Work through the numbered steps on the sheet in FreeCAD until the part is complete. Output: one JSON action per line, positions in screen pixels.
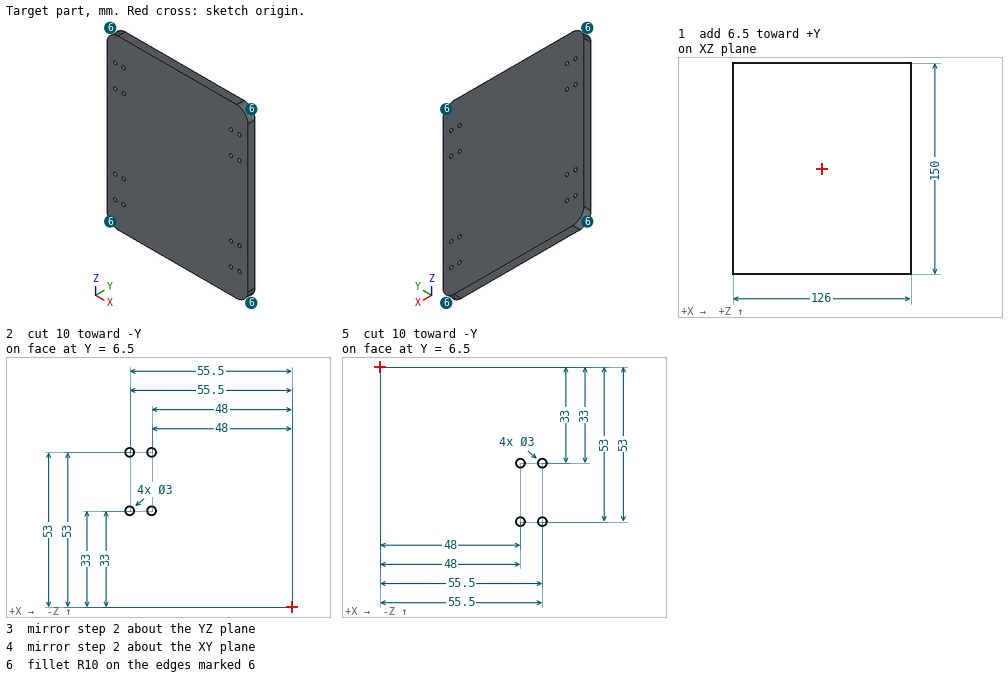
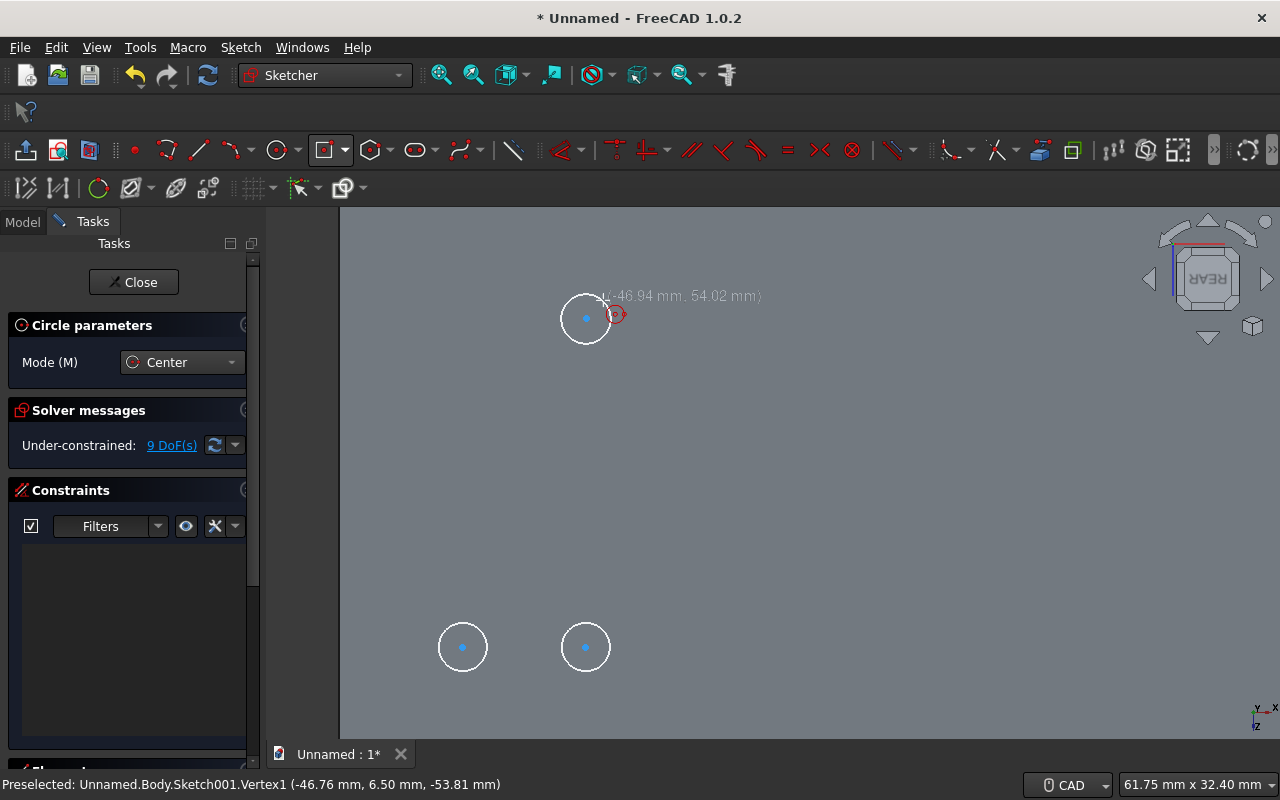
{"action": "left_click", "coordinate": [463, 318]}
{"action": "left_click", "coordinate": [480, 300]}
{"action": "key", "text": "Escape"}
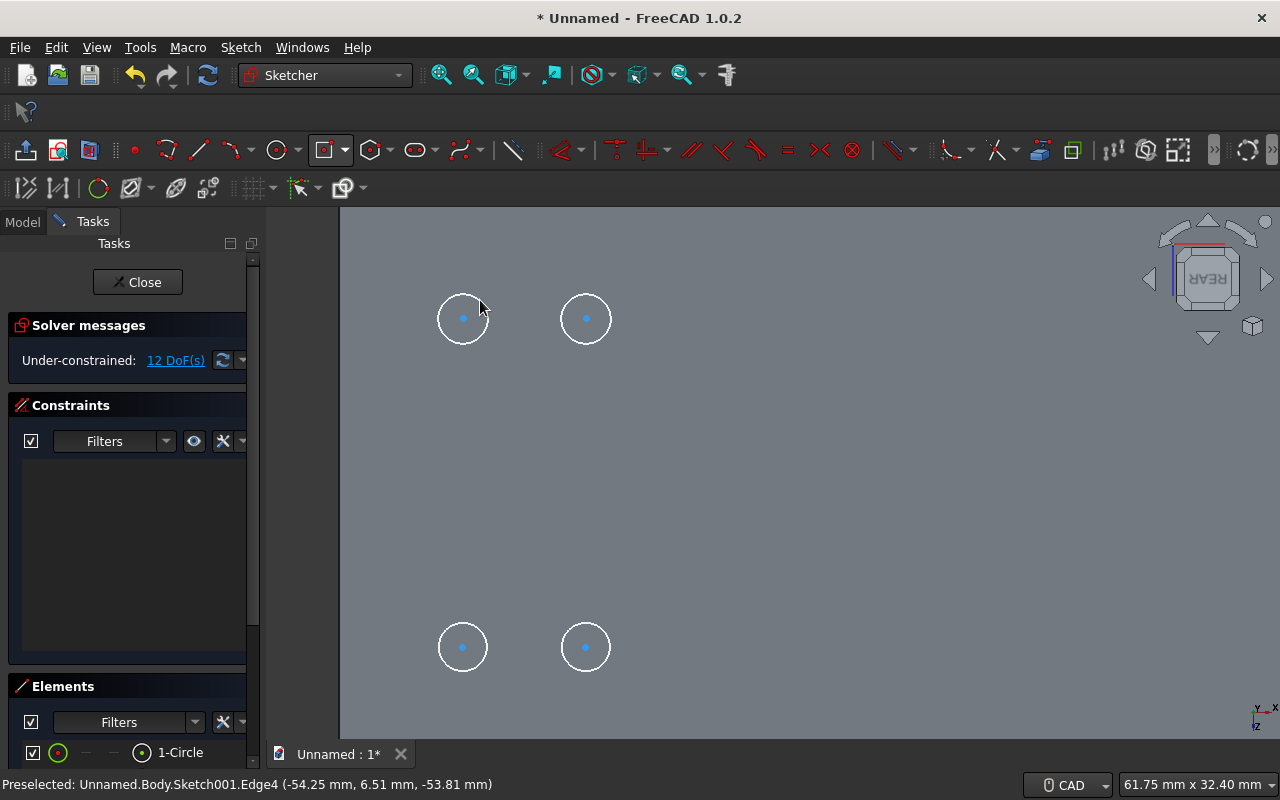
{"action": "left_click", "coordinate": [480, 630]}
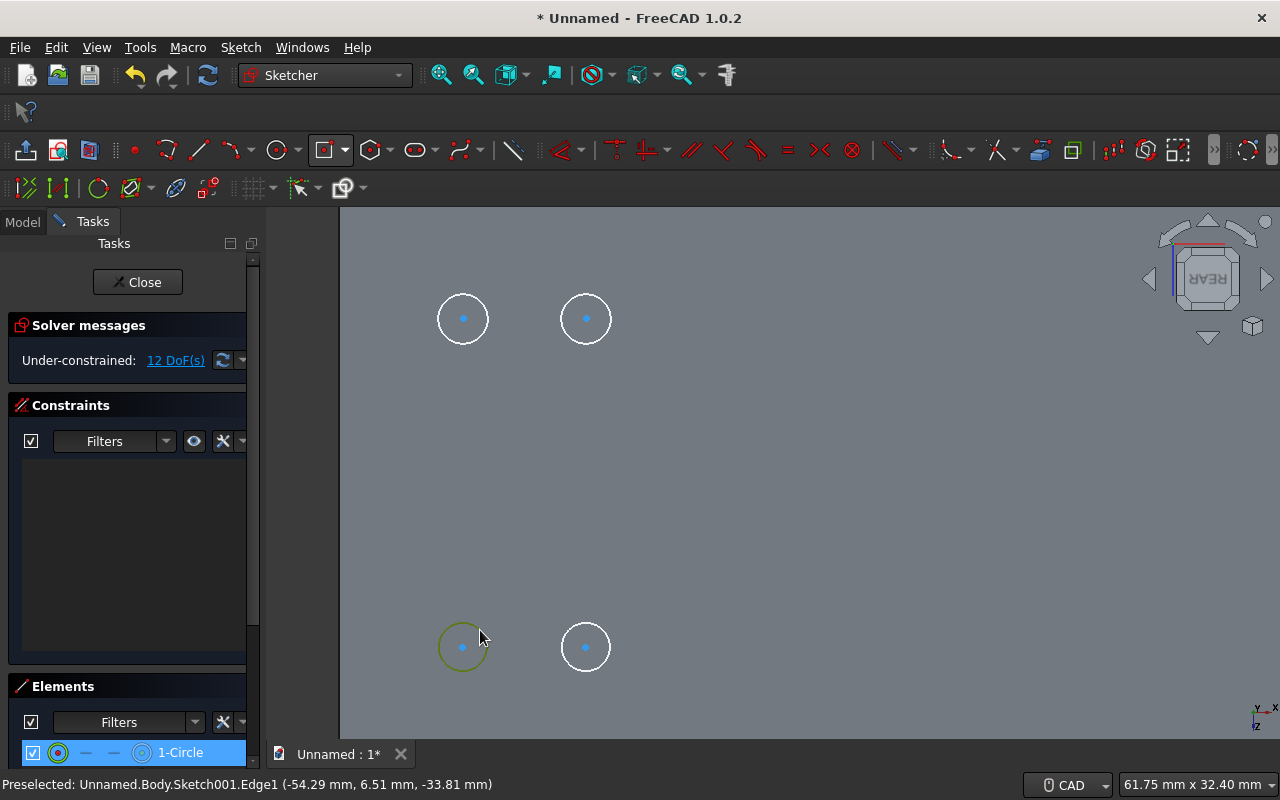
{"action": "left_click", "coordinate": [603, 630]}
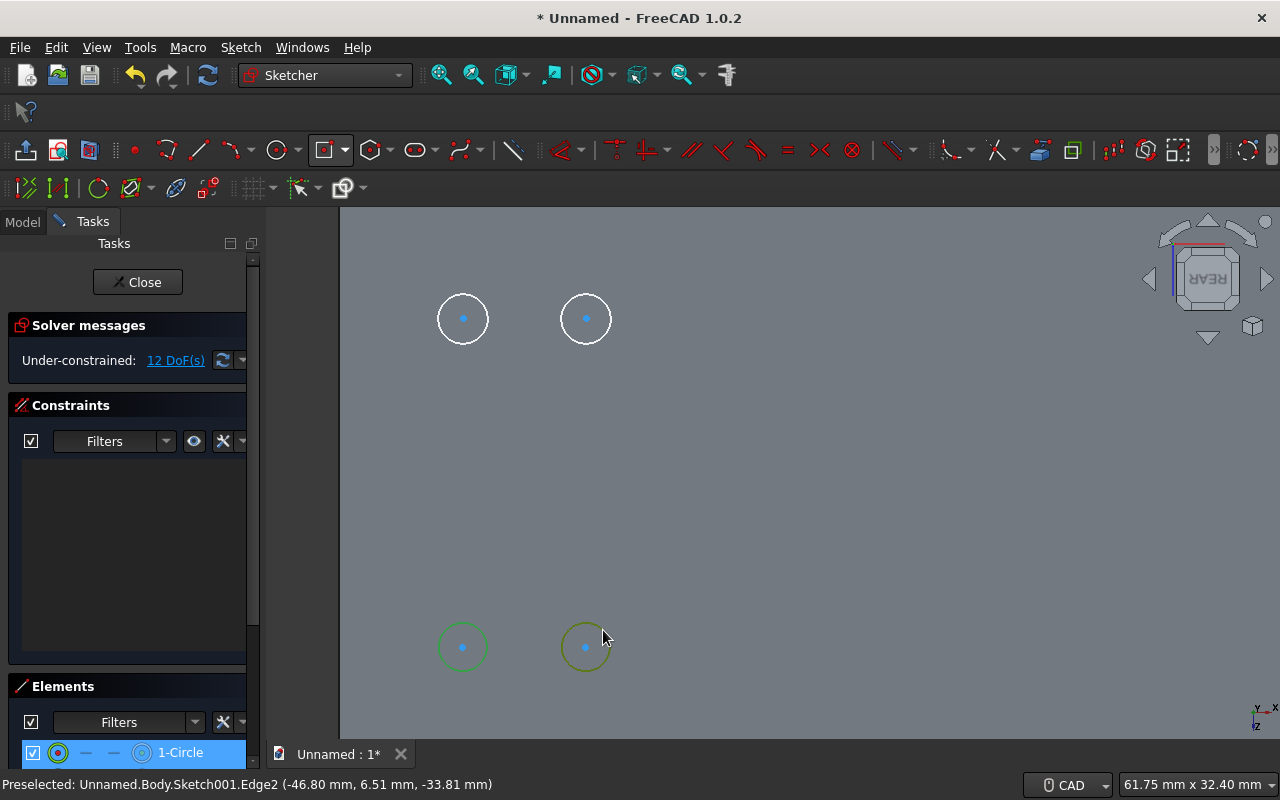
{"action": "left_click", "coordinate": [603, 301]}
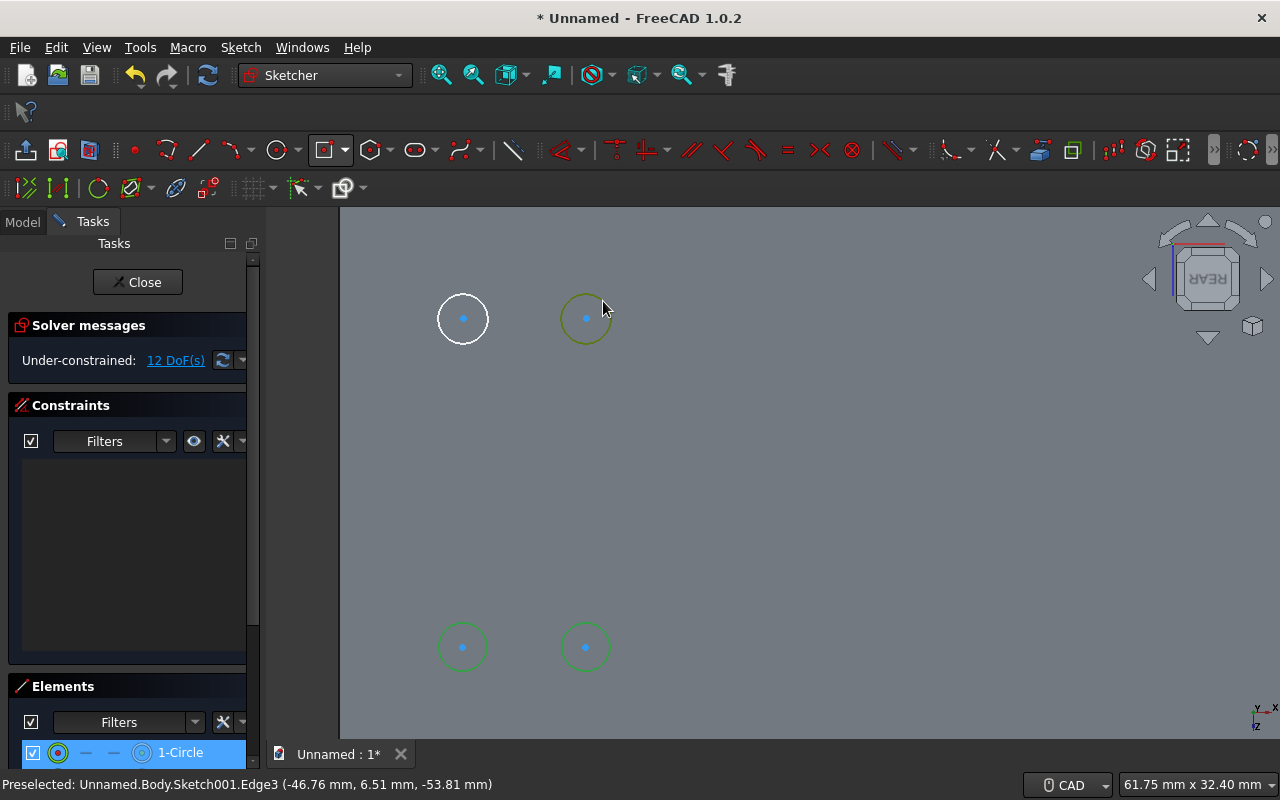
{"action": "left_click", "coordinate": [480, 301]}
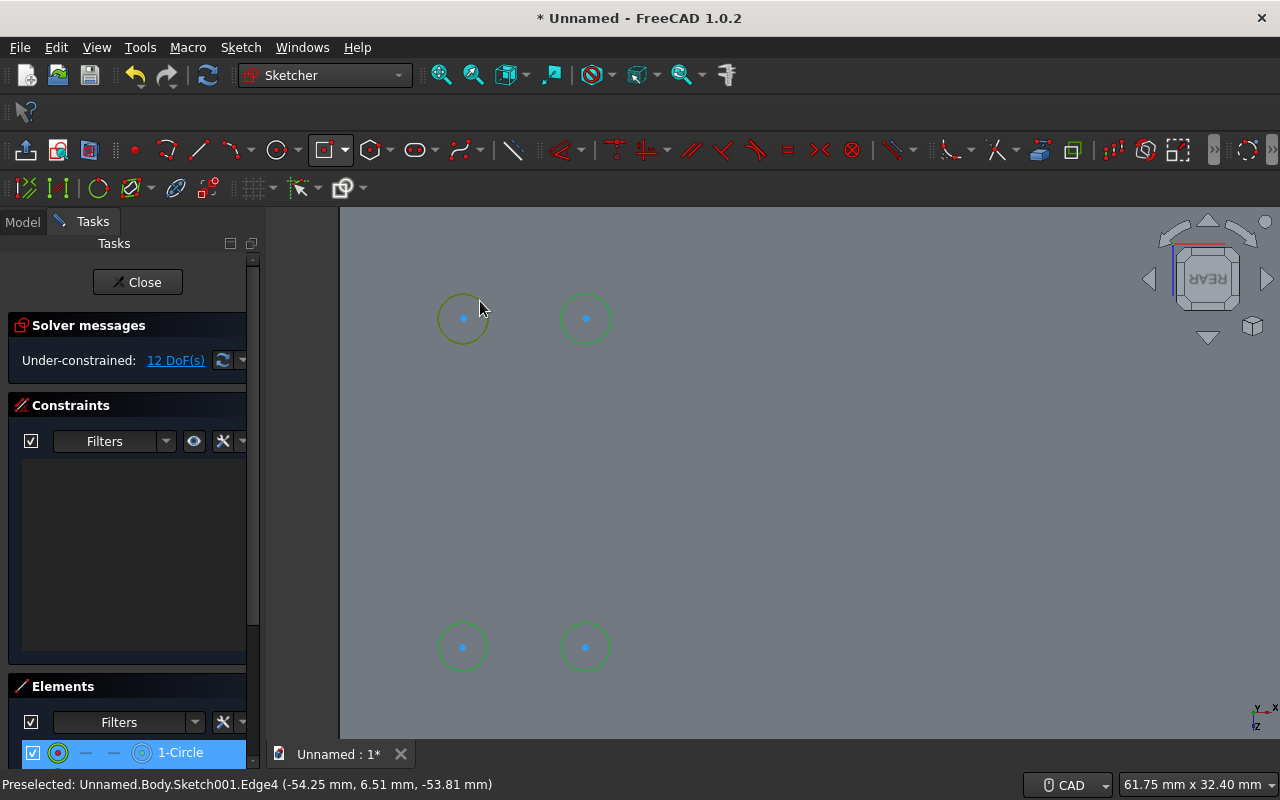
{"action": "key", "text": "e"}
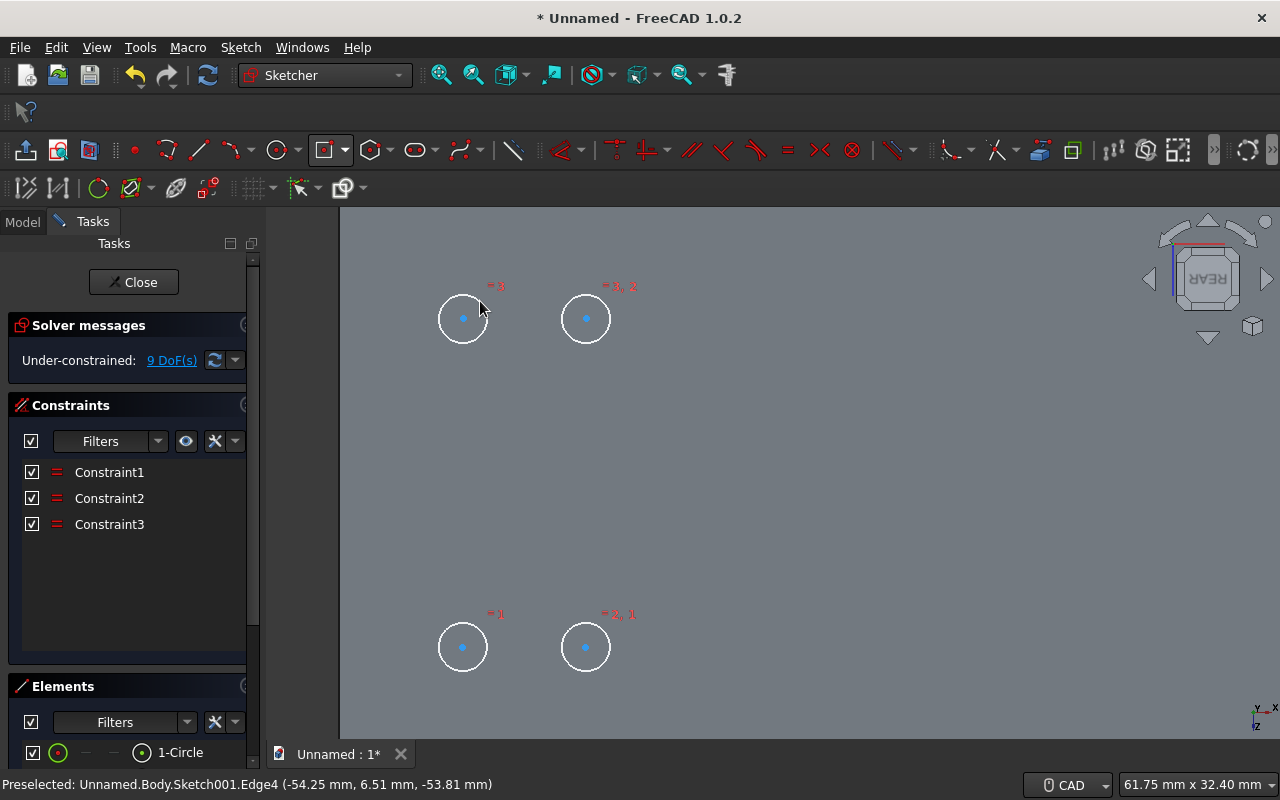
{"action": "left_click", "coordinate": [560, 150]}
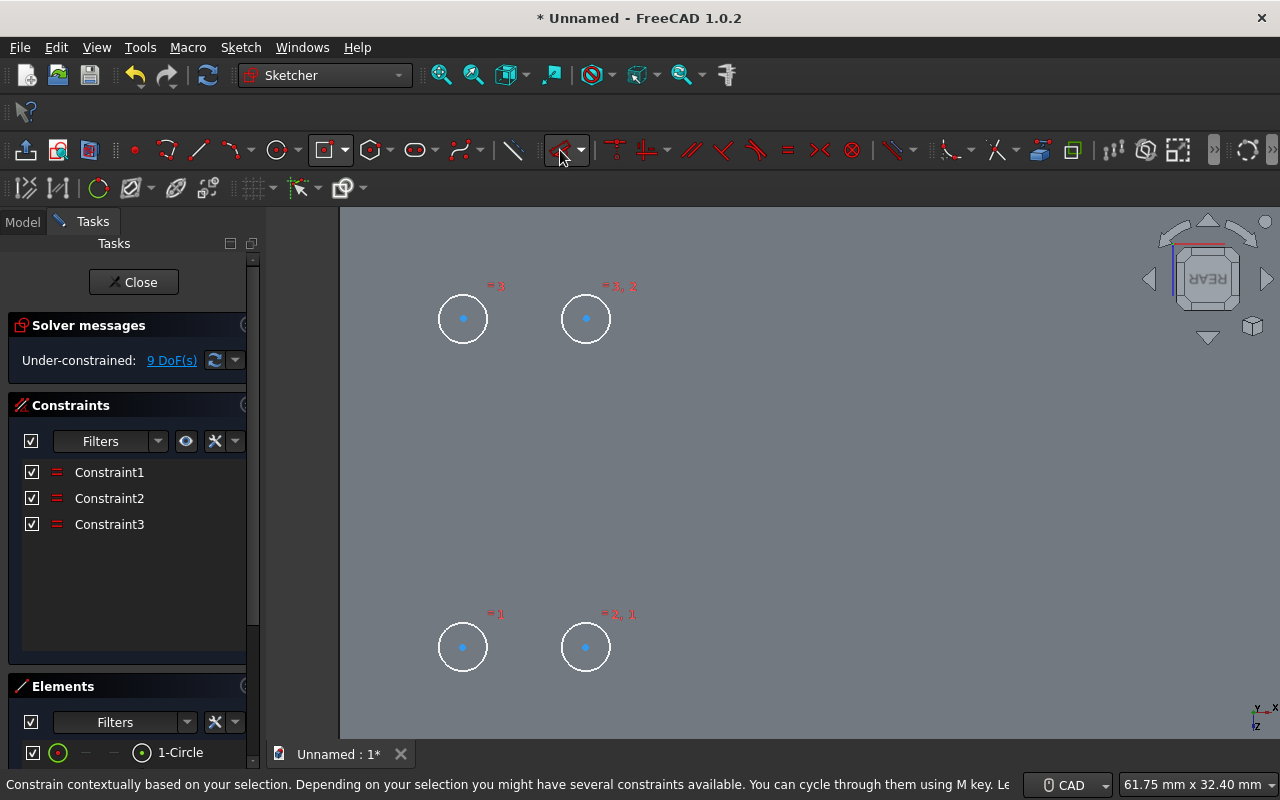
{"action": "left_click", "coordinate": [480, 630]}
{"action": "left_click", "coordinate": [503, 607]}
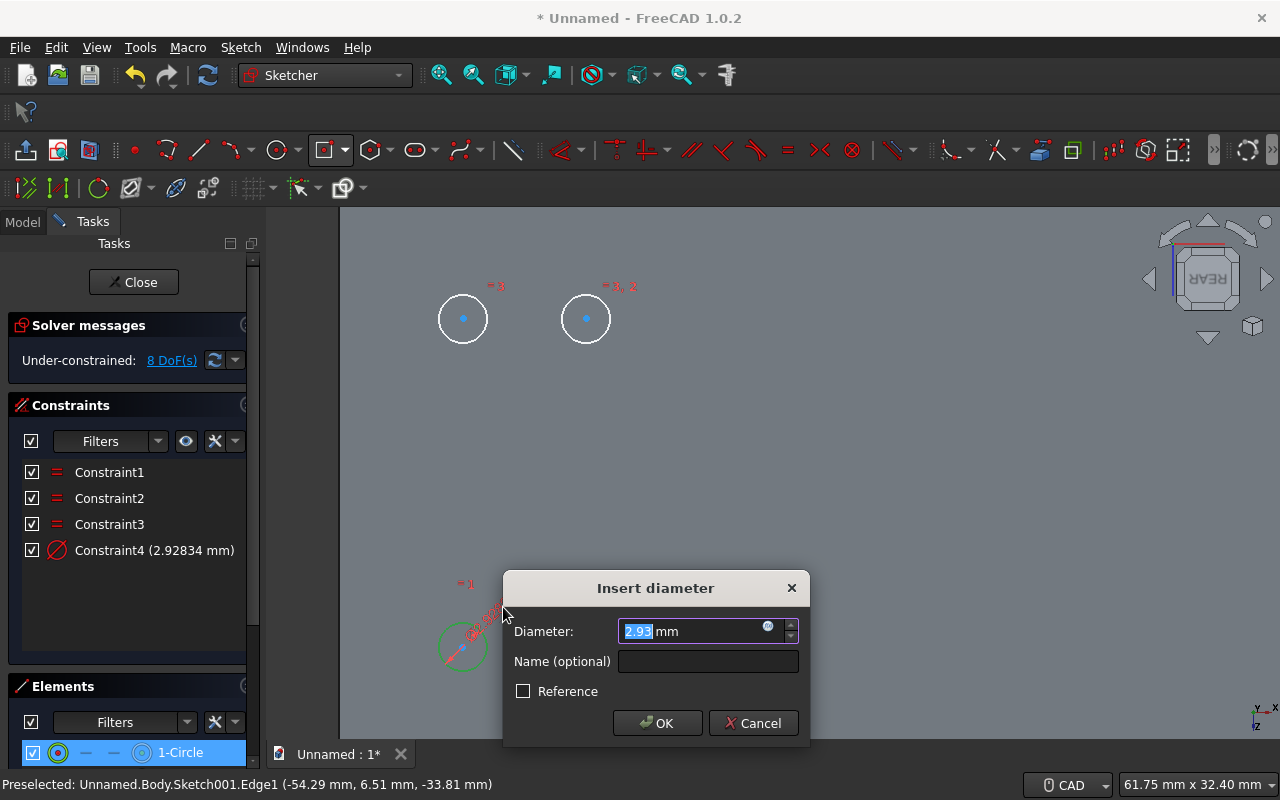
{"action": "type", "text": "3"}
{"action": "key", "text": "Return"}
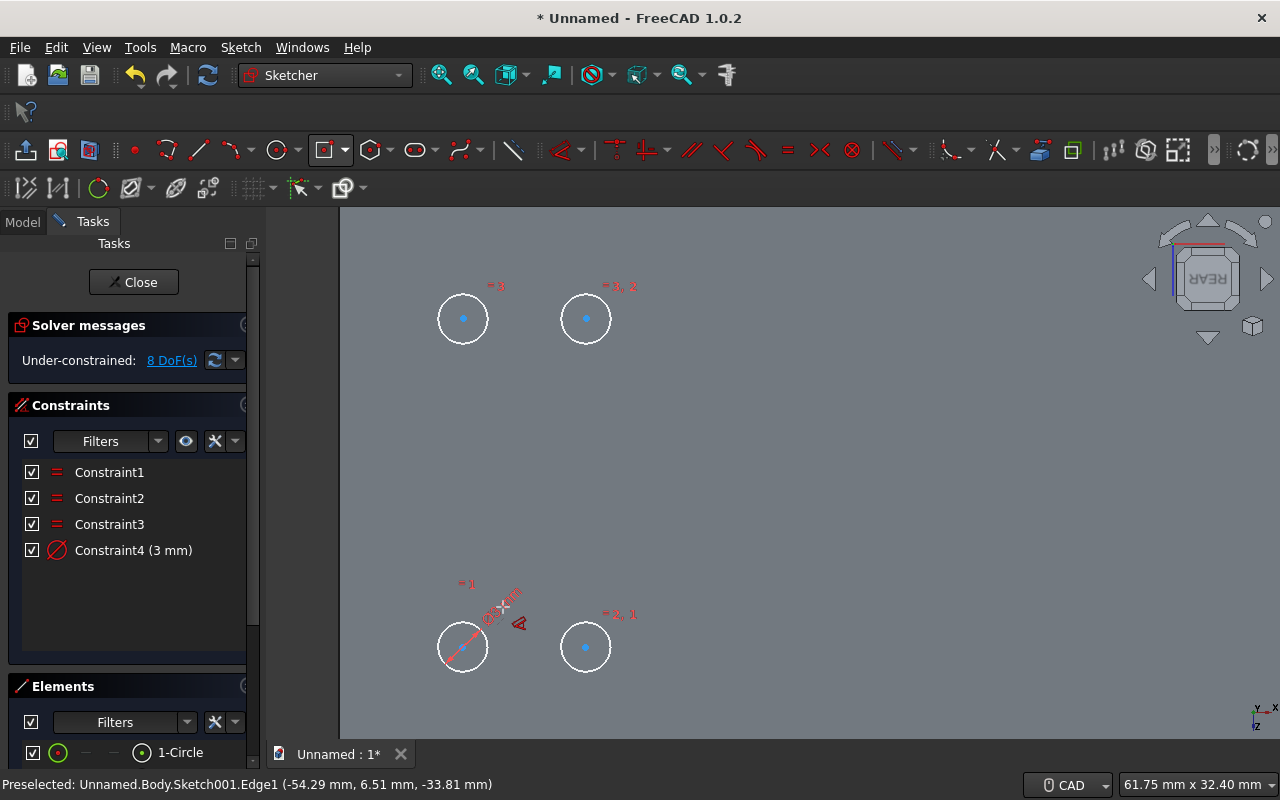
{"action": "left_click", "coordinate": [463, 647]}
{"action": "left_click", "coordinate": [429, 679]}